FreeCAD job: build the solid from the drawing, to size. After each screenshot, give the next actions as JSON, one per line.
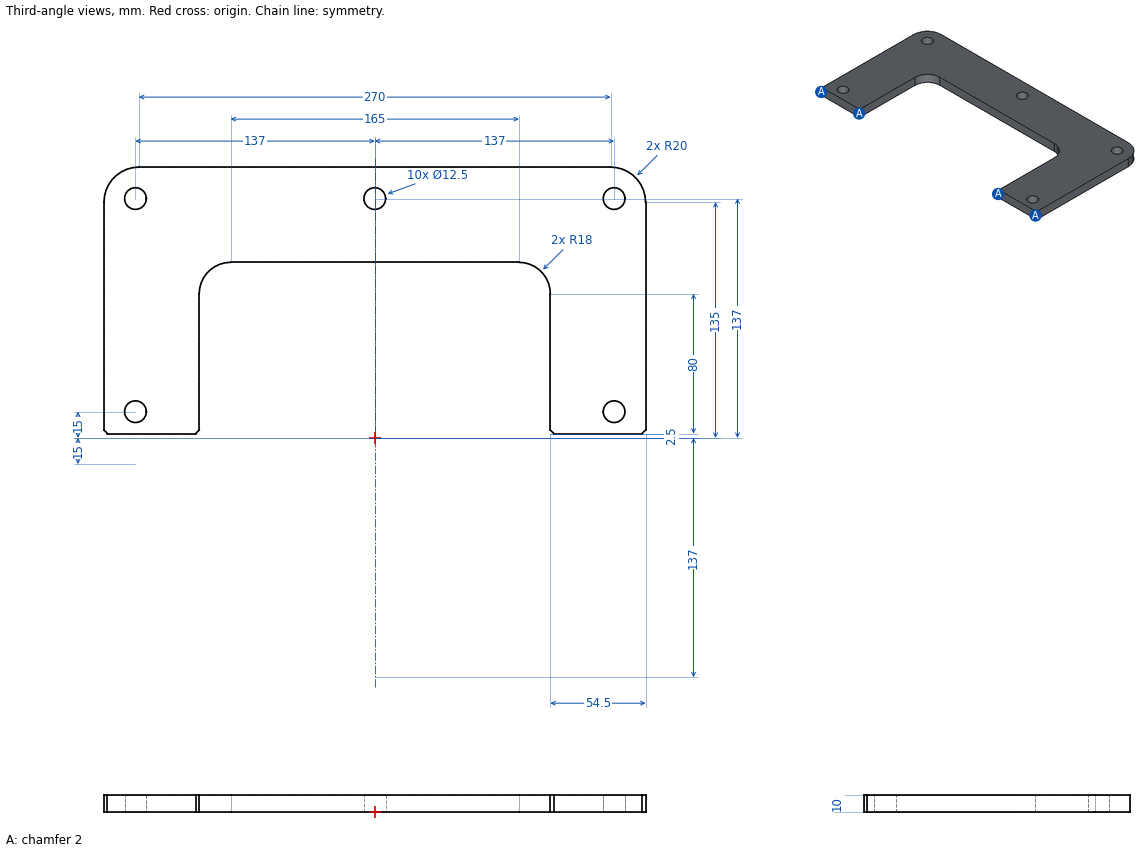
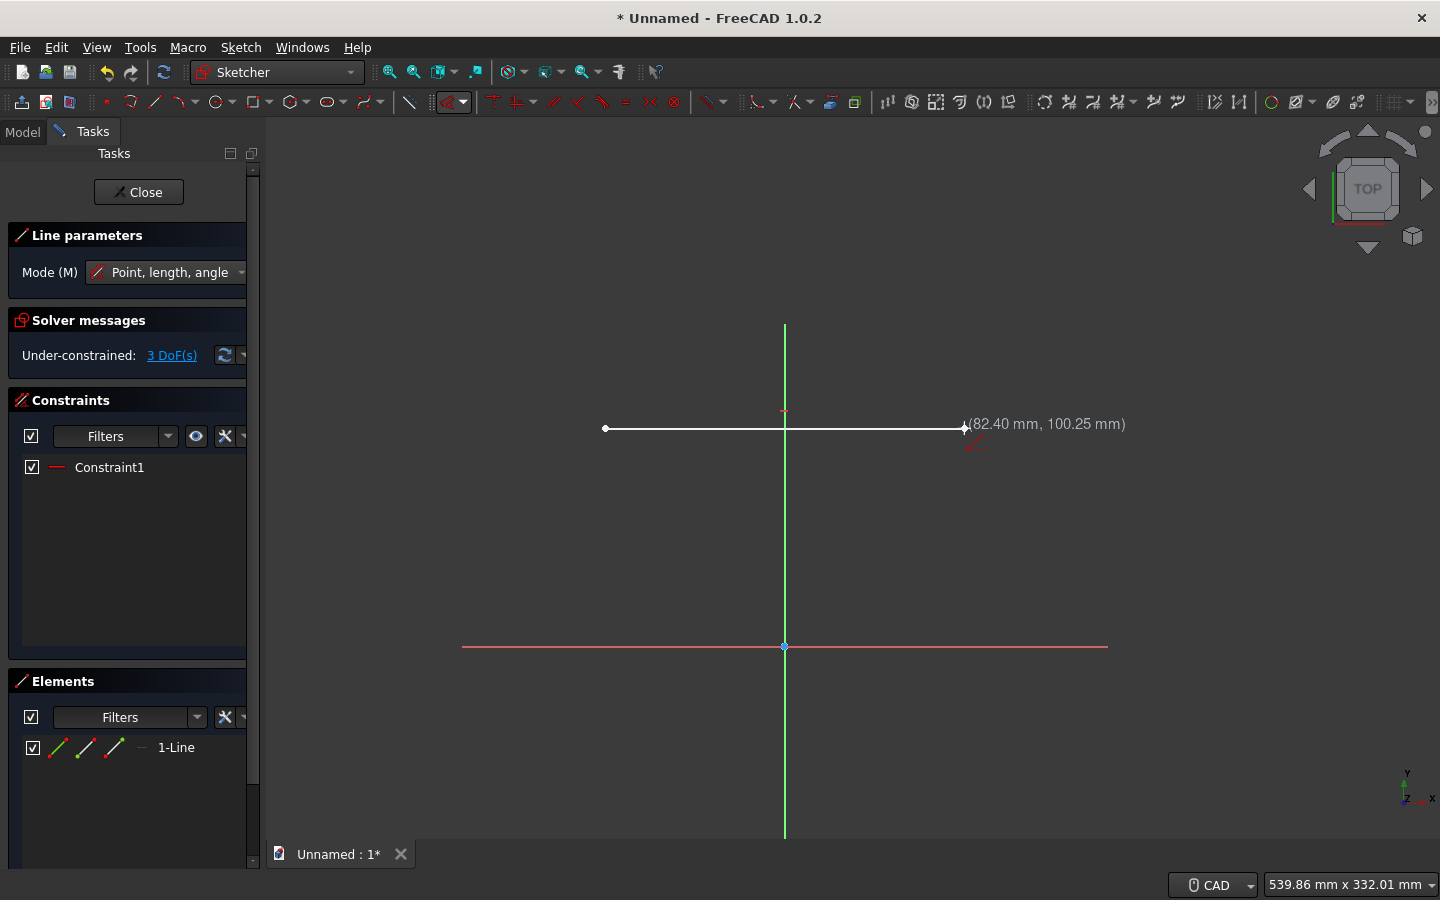
{"action": "left_click", "coordinate": [132, 102]}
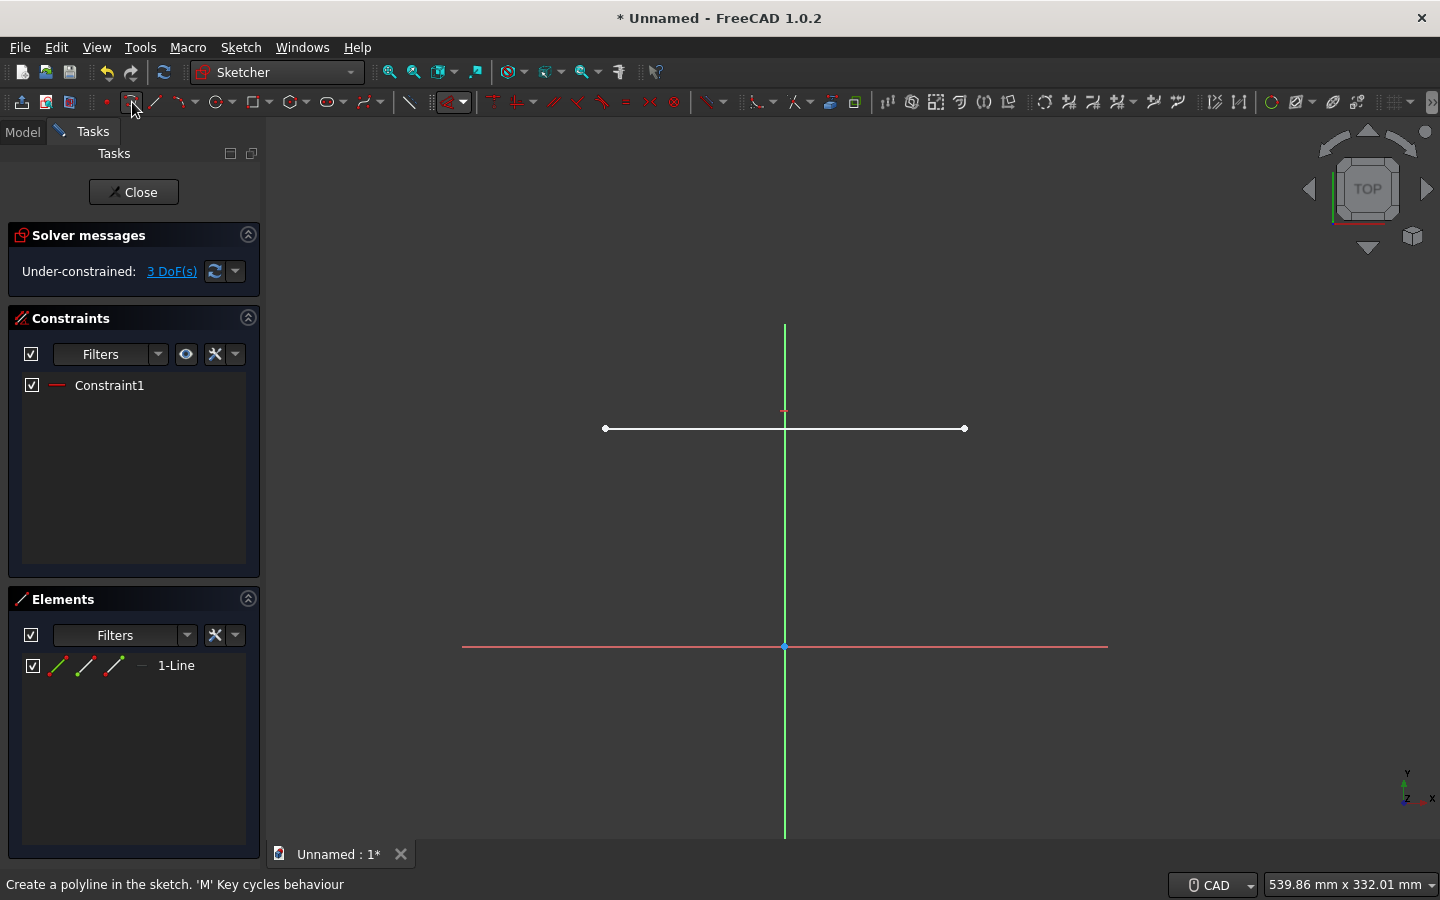
{"action": "left_click", "coordinate": [1003, 468]}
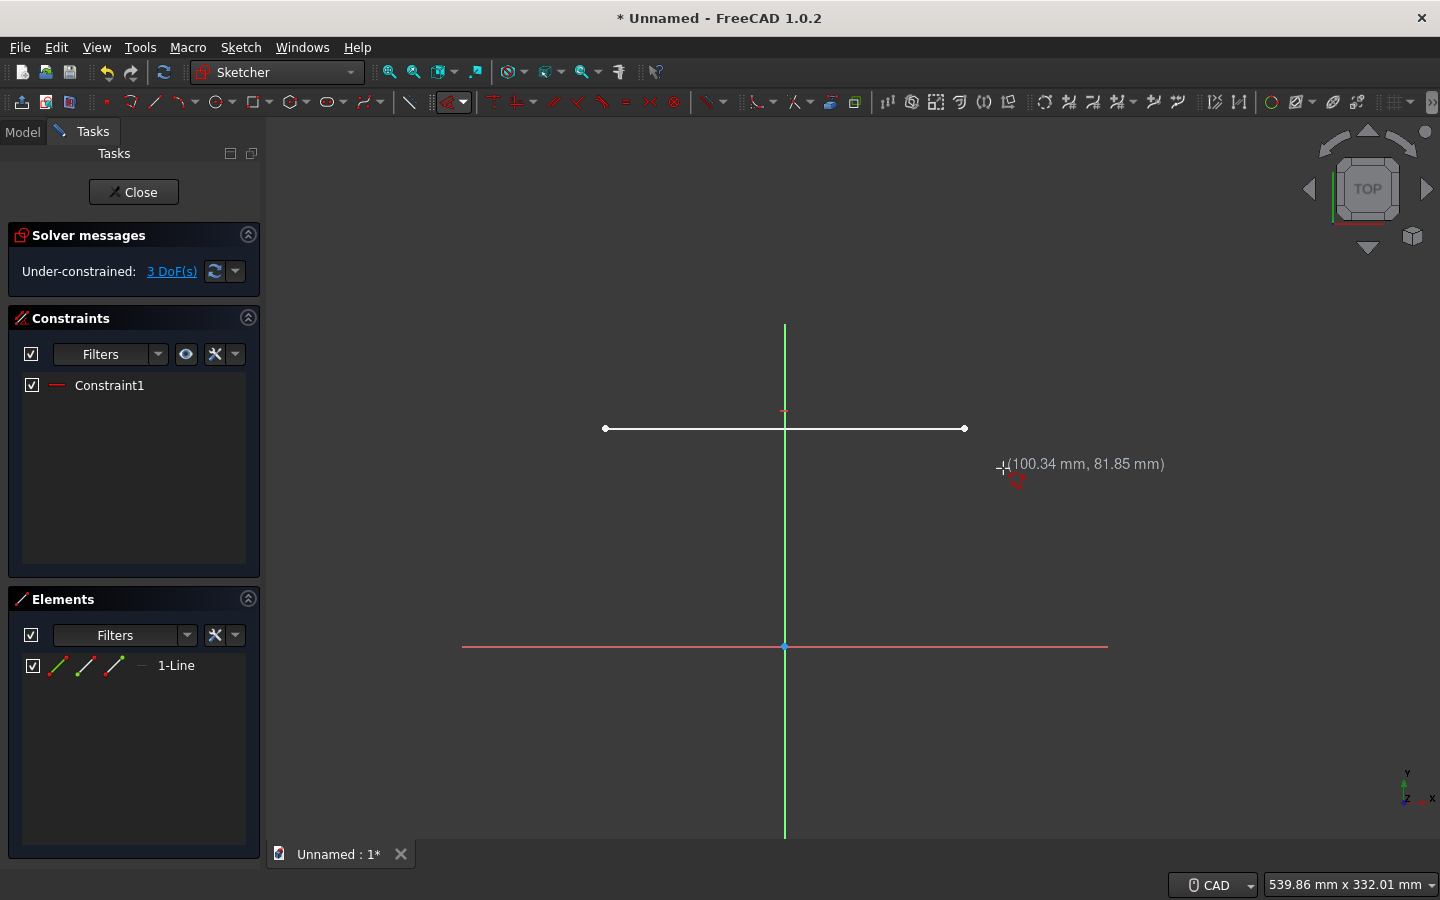
{"action": "scroll", "coordinate": [1003, 642], "scroll_direction": "up", "scroll_amount": 6}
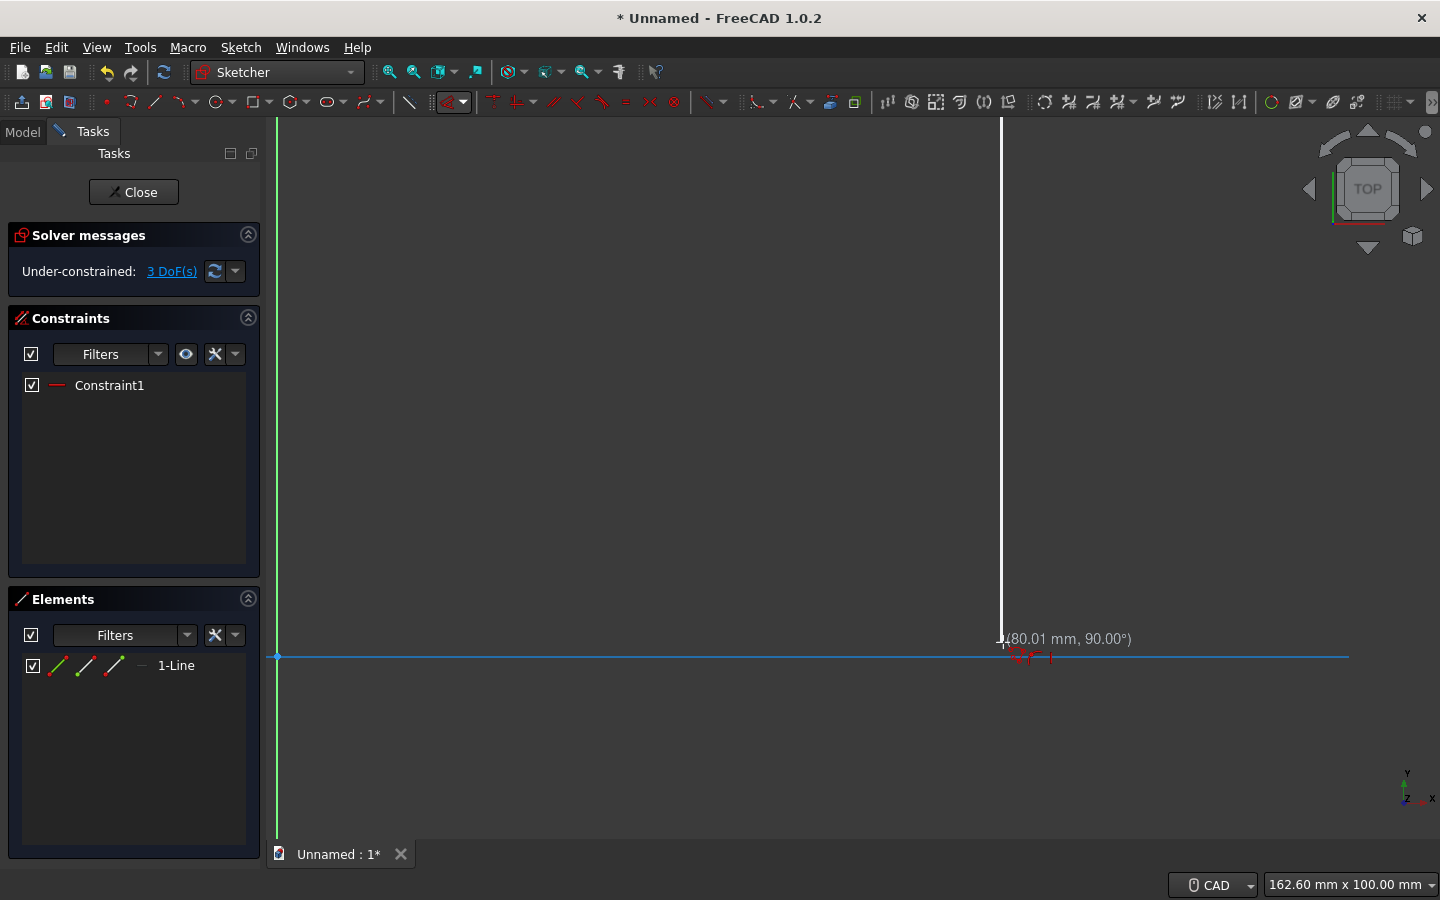
{"action": "left_click", "coordinate": [1002, 639]}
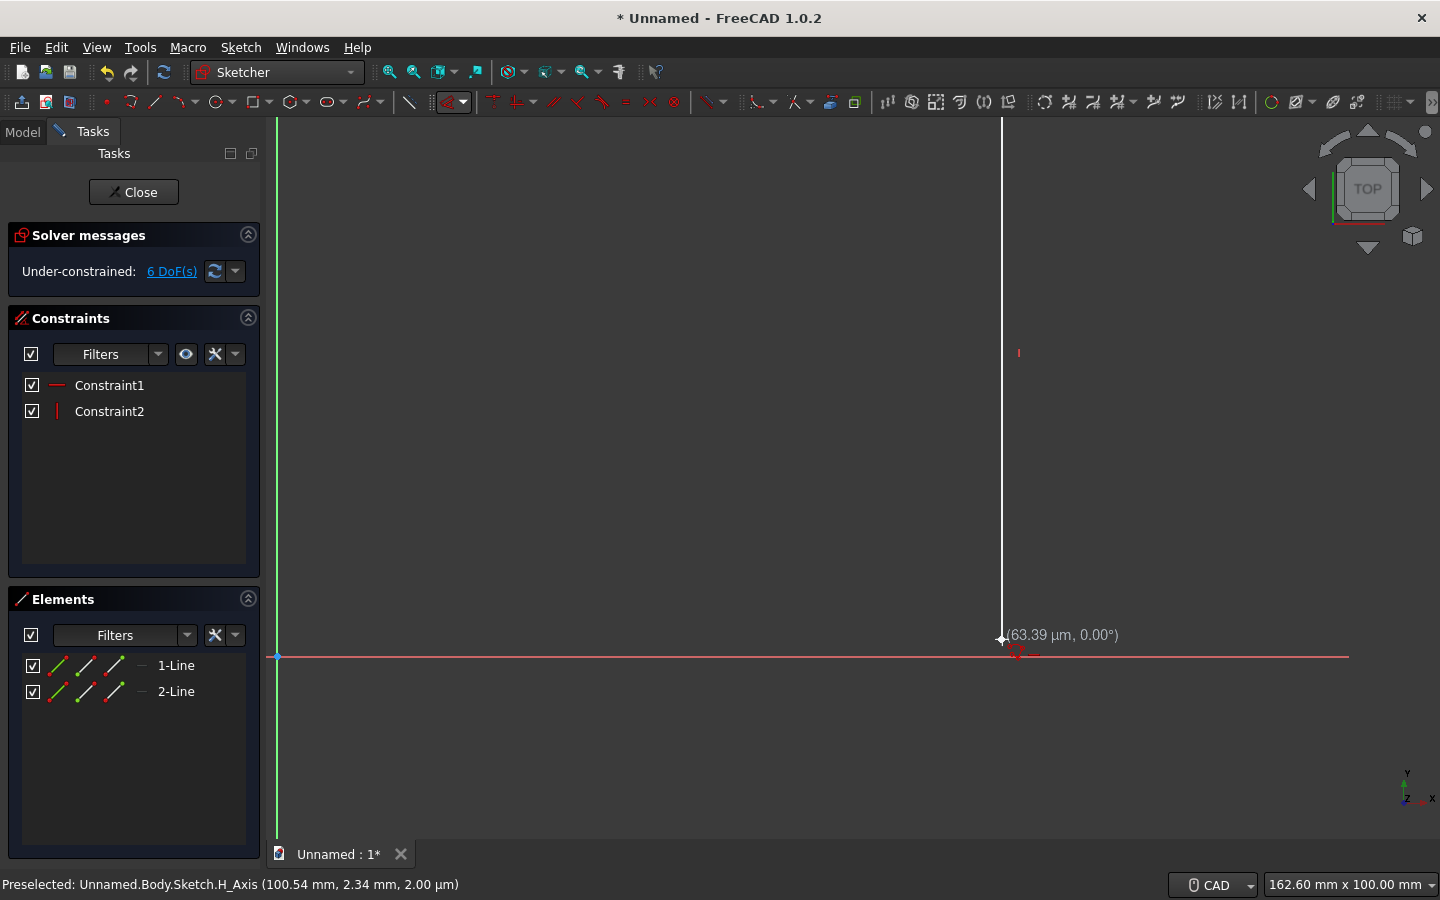
{"action": "scroll", "coordinate": [1003, 642], "scroll_direction": "down", "scroll_amount": 6}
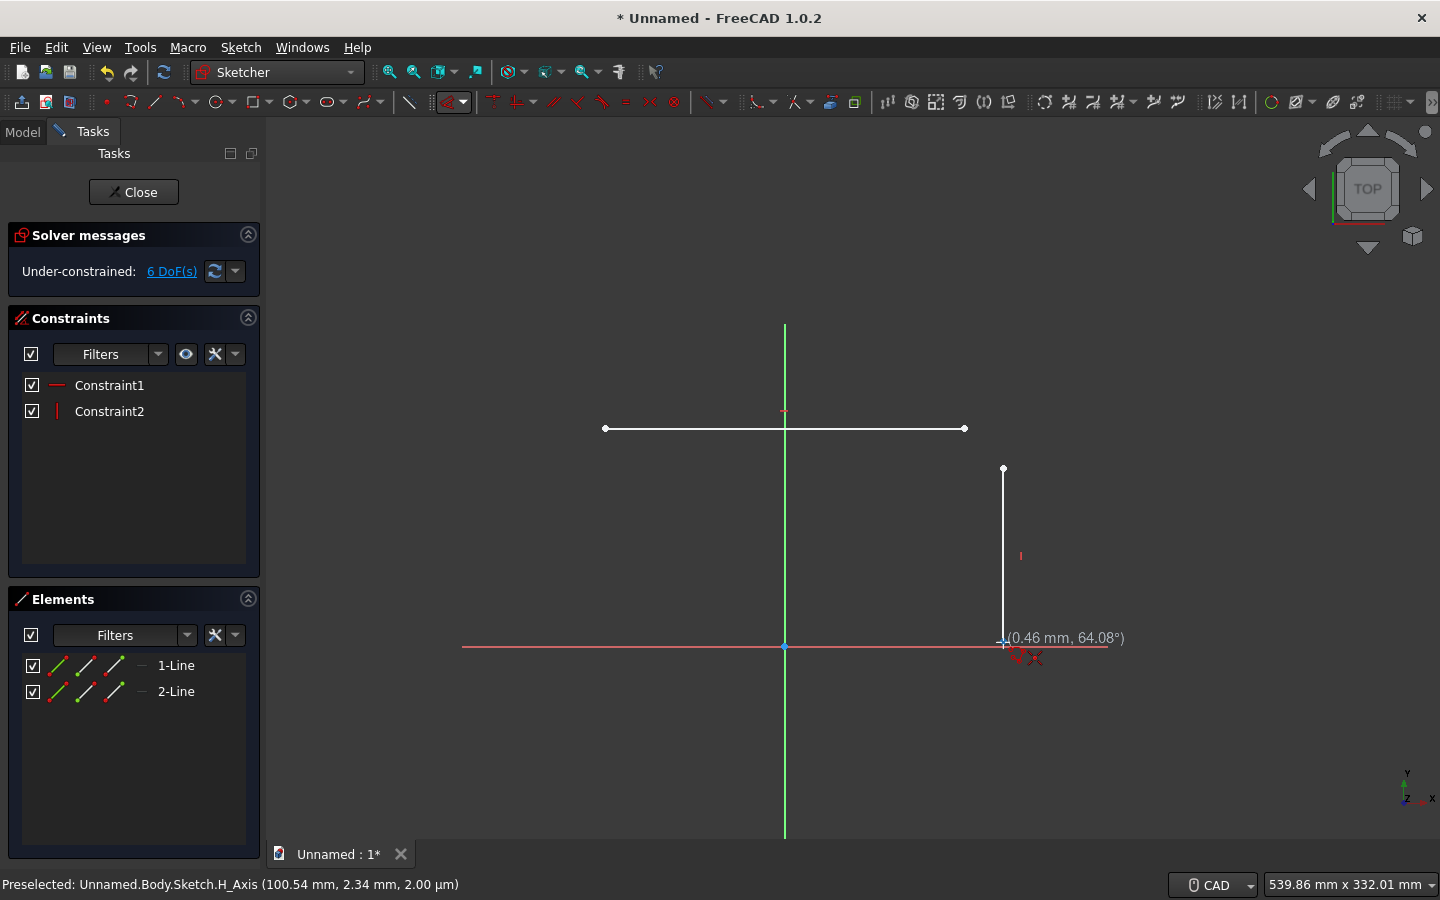
{"action": "scroll", "coordinate": [1122, 642], "scroll_direction": "up", "scroll_amount": 6}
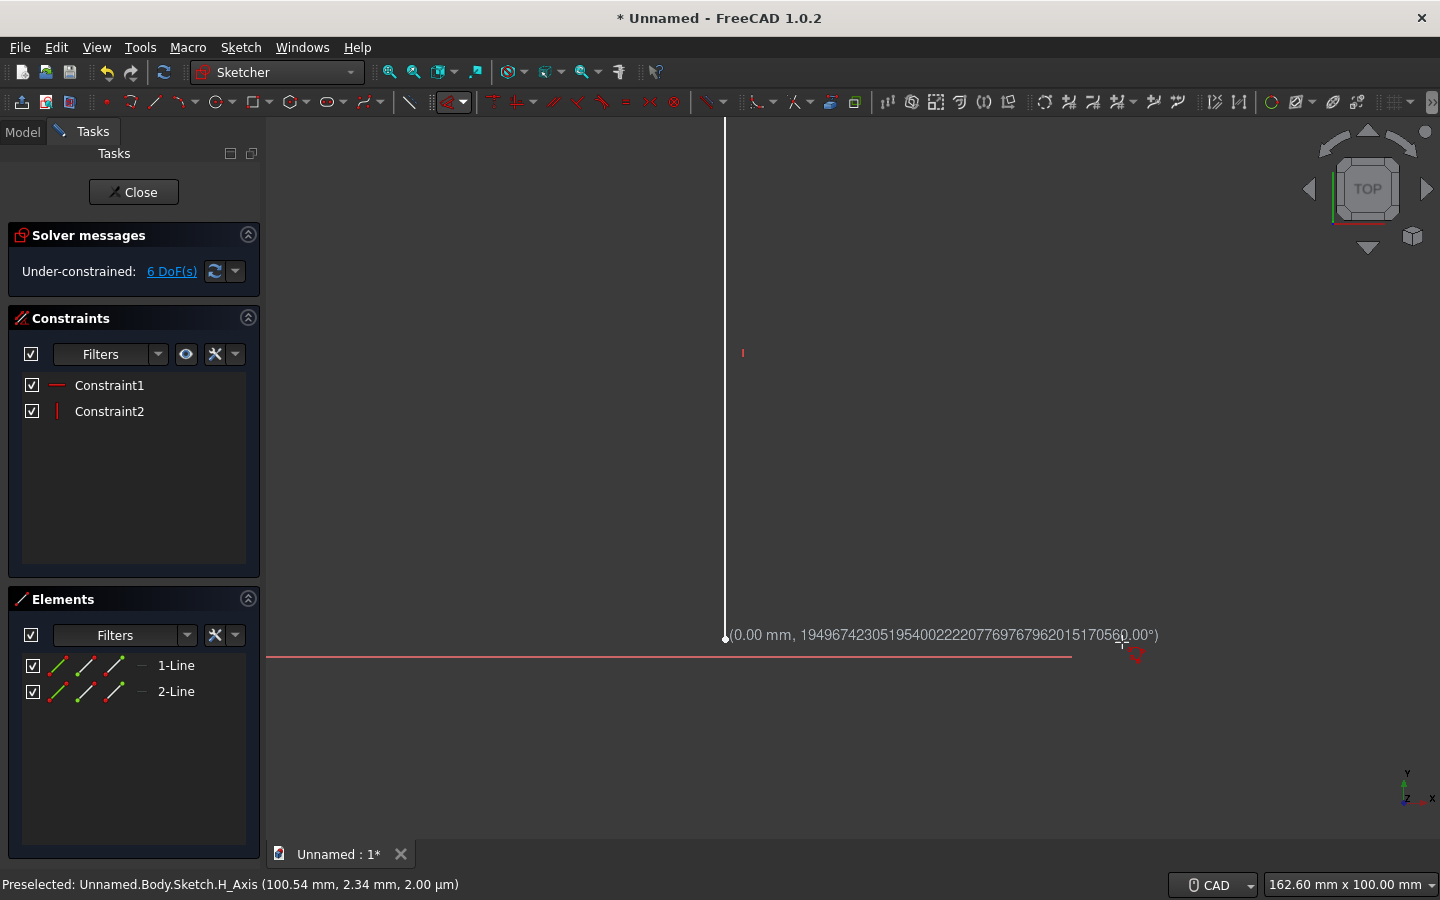
{"action": "left_click", "coordinate": [1120, 639]}